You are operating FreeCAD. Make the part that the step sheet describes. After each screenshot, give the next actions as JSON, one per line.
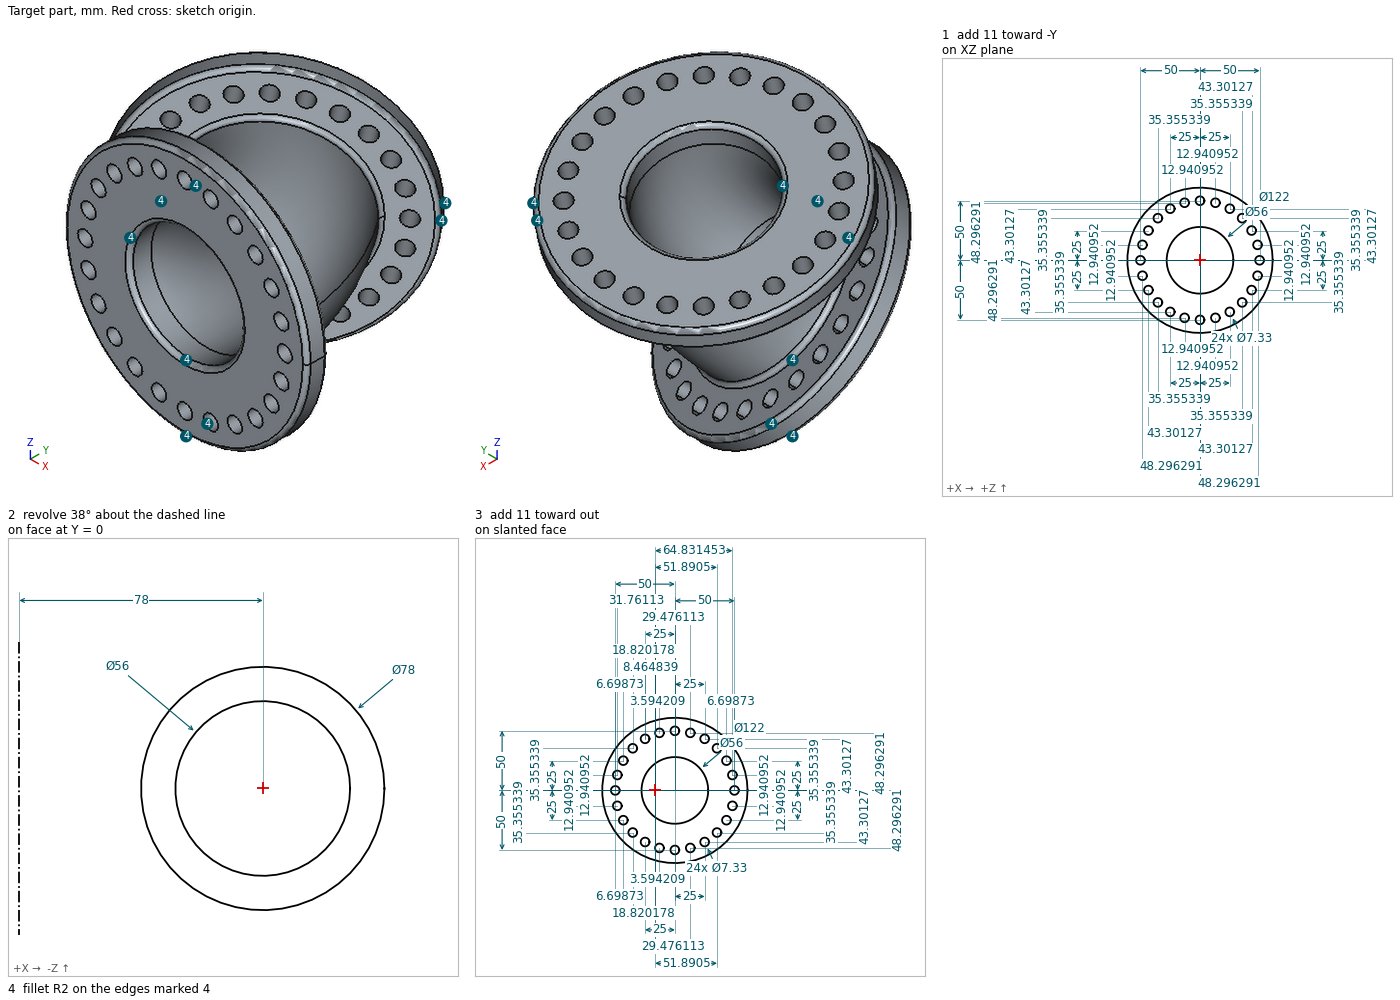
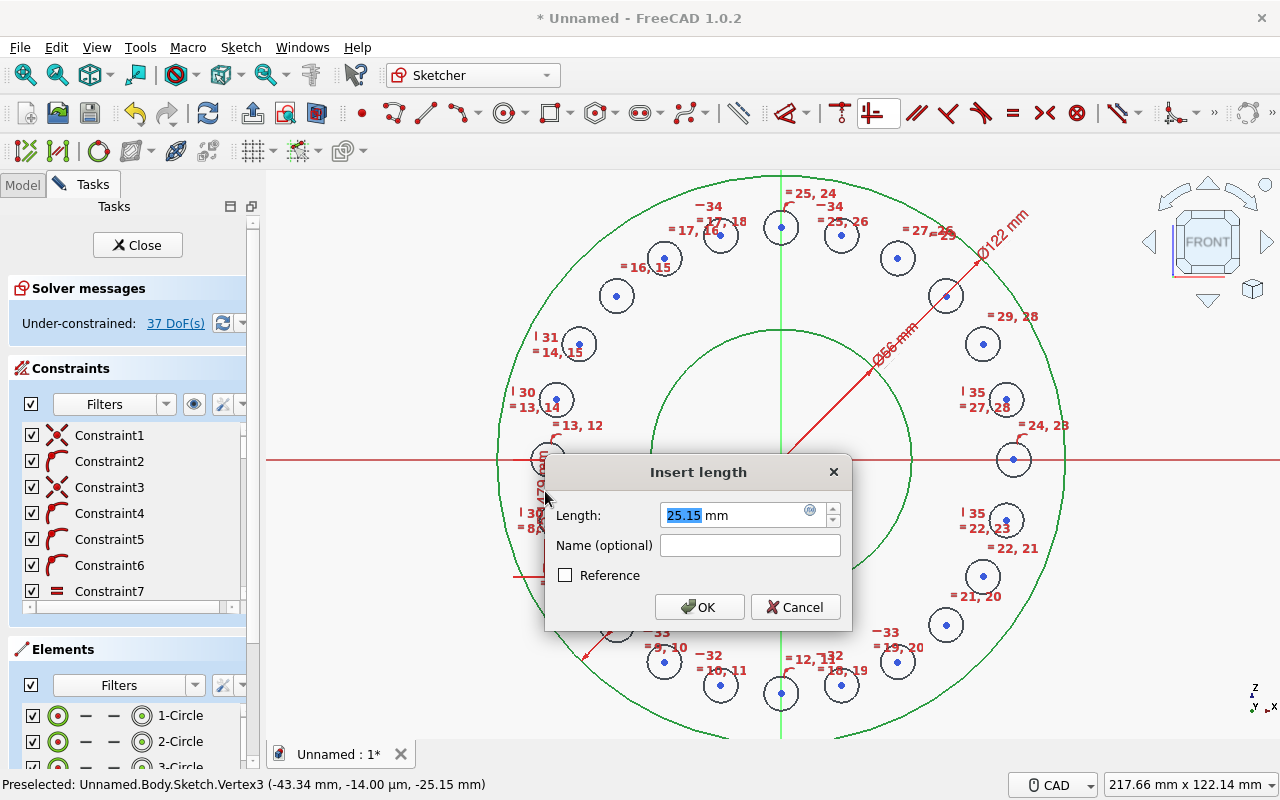
{"action": "type", "text": "25"}
{"action": "key", "text": "Return"}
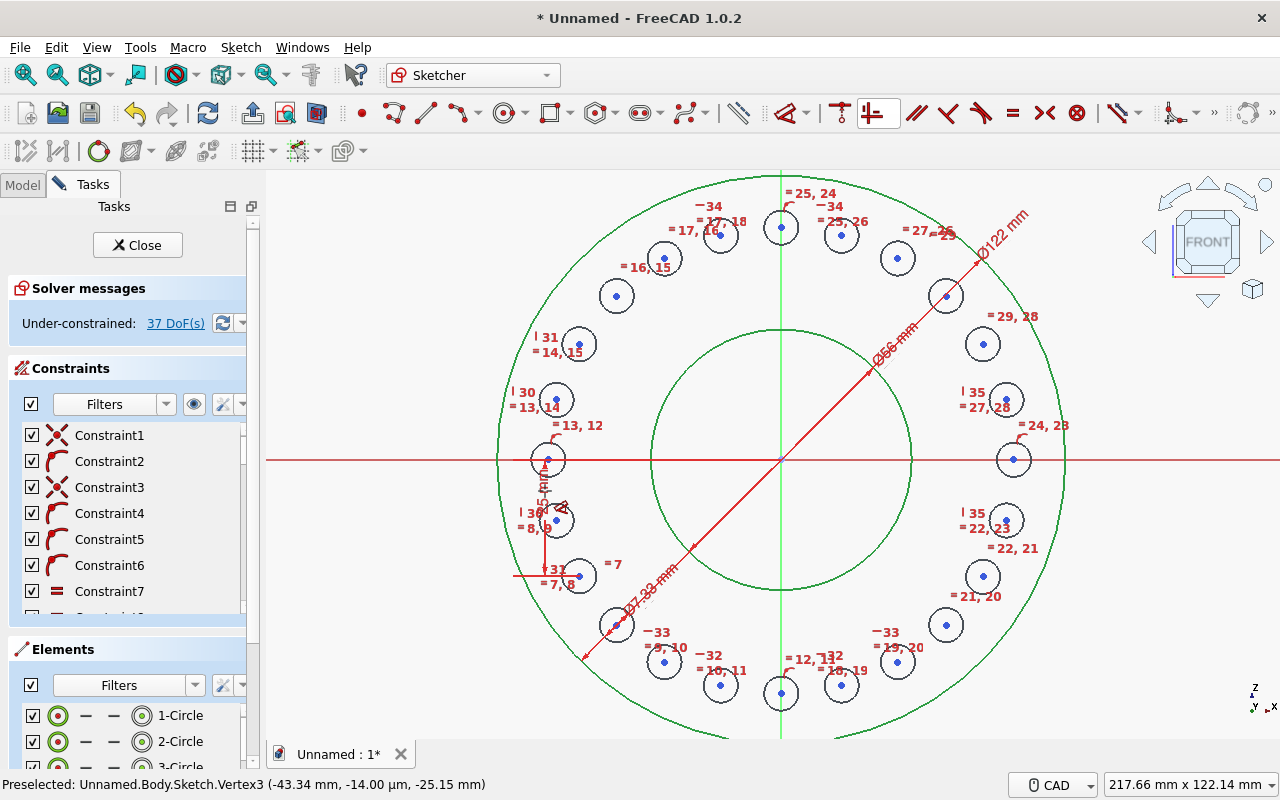
{"action": "left_click", "coordinate": [664, 662]}
{"action": "left_click", "coordinate": [750, 696]}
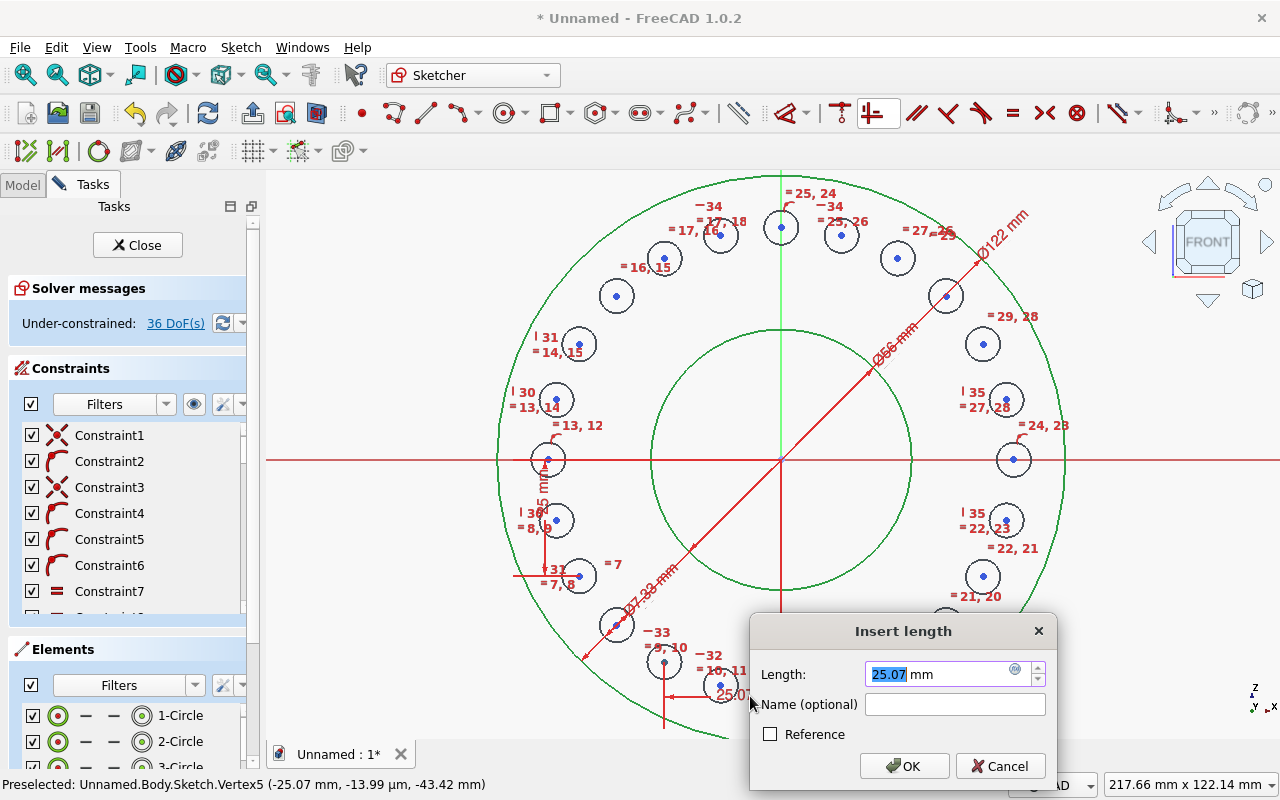
{"action": "type", "text": "25"}
{"action": "key", "text": "Return"}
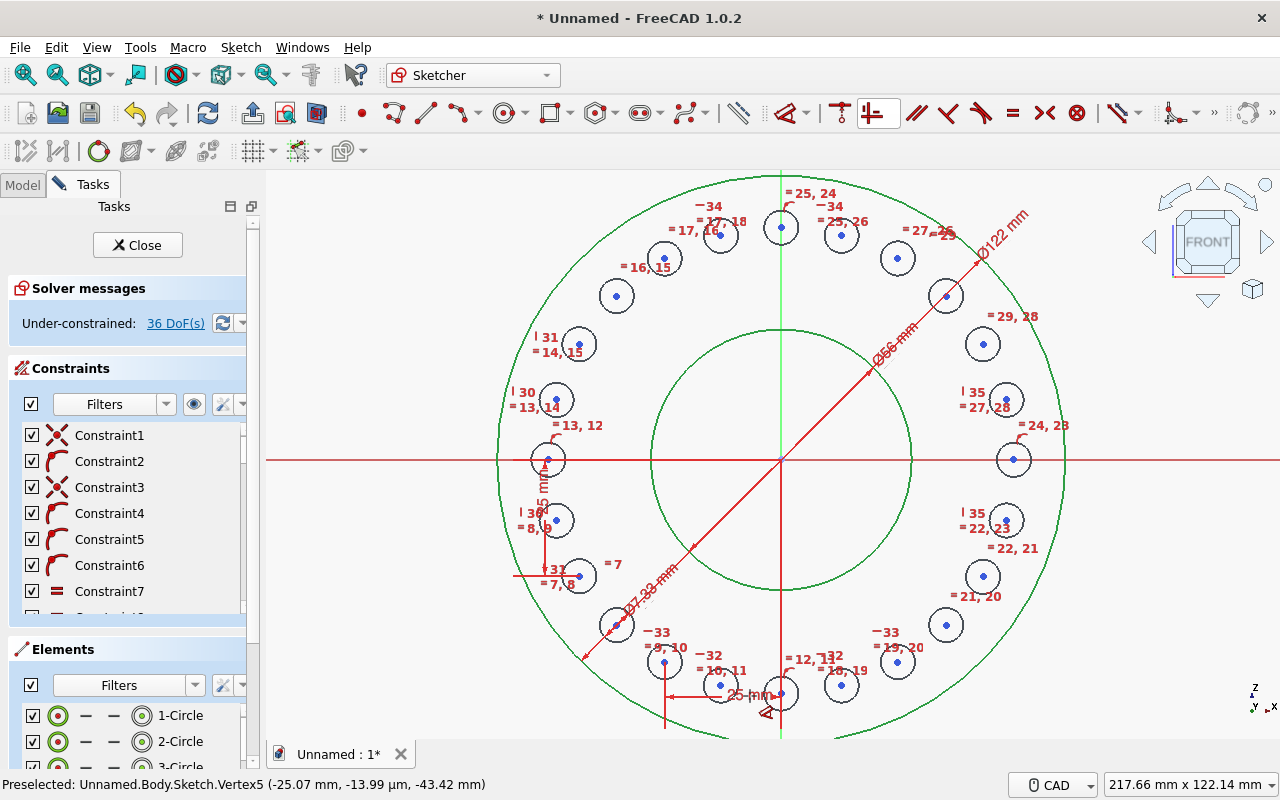
{"action": "left_click", "coordinate": [781, 694]}
{"action": "left_click", "coordinate": [815, 523]}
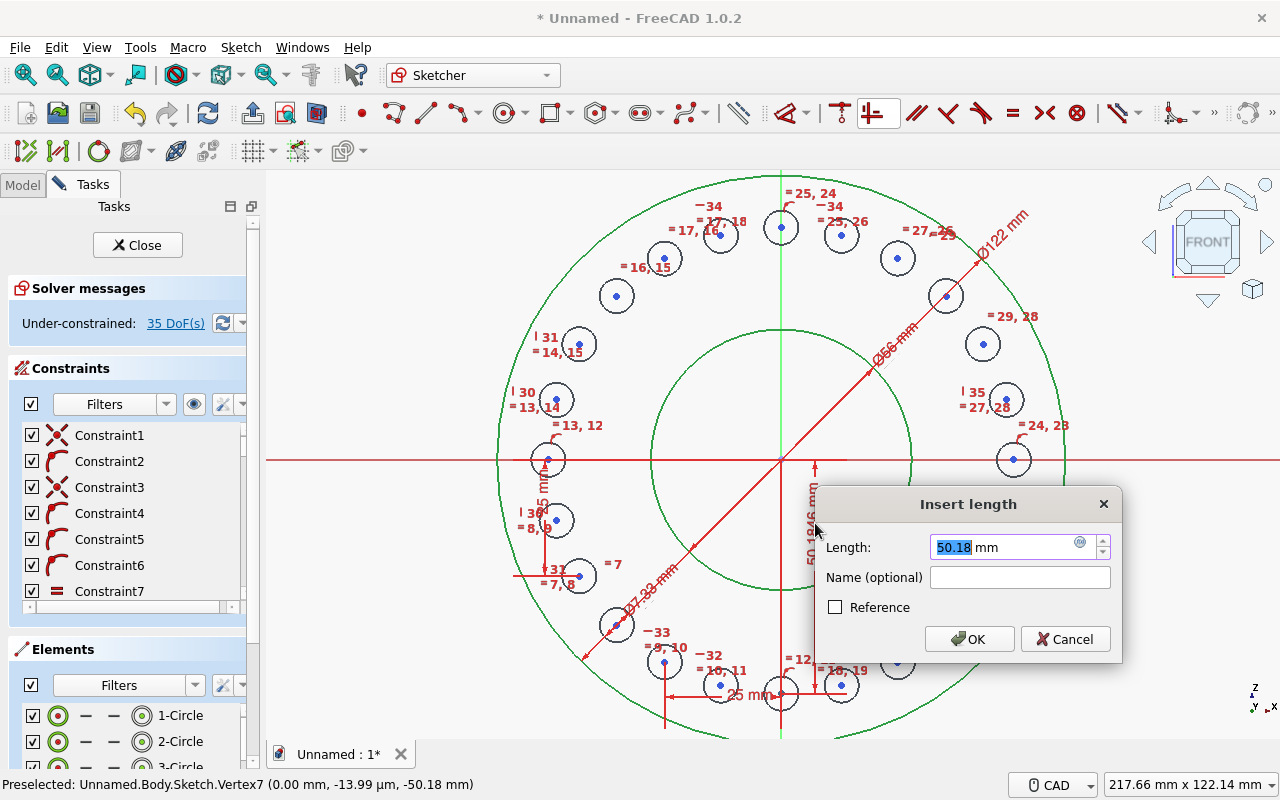
{"action": "type", "text": "50"}
{"action": "key", "text": "Return"}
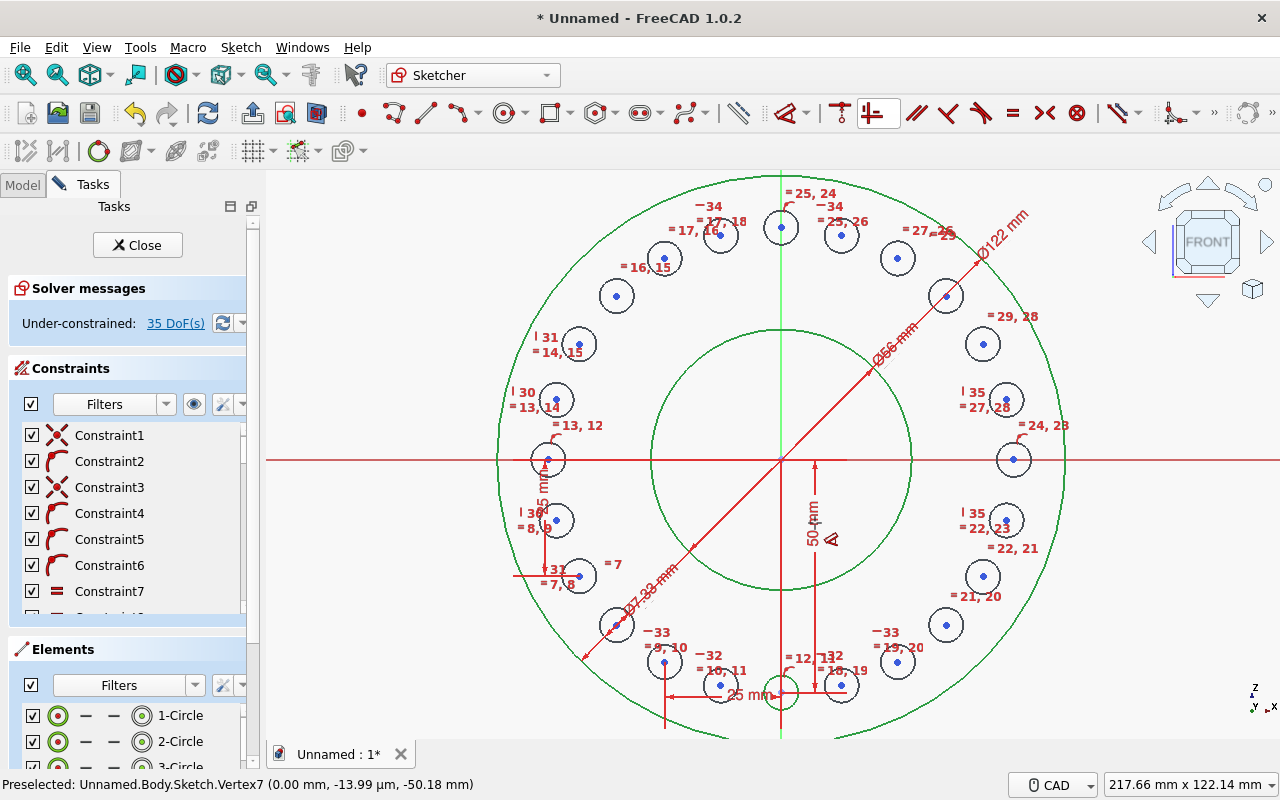
{"action": "left_click", "coordinate": [548, 460]}
{"action": "left_click", "coordinate": [718, 494]}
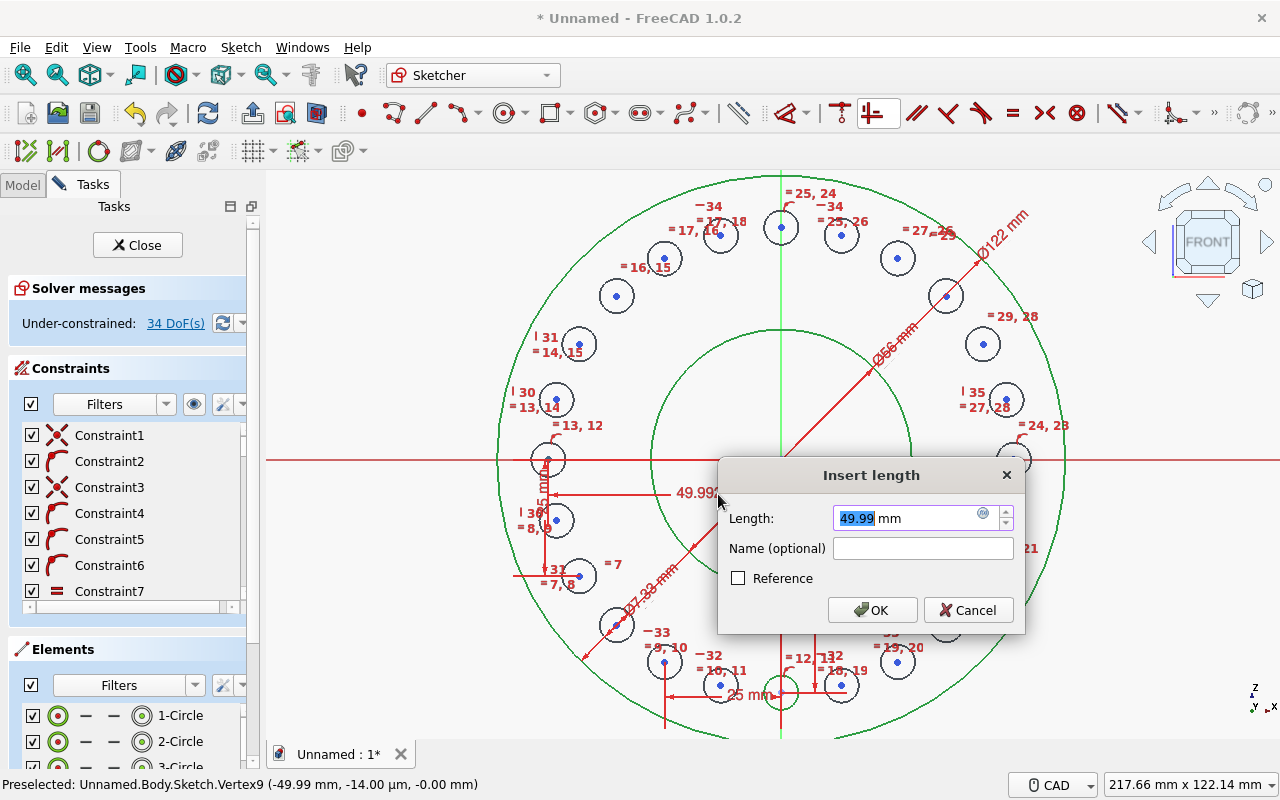
{"action": "type", "text": "50"}
{"action": "key", "text": "Return"}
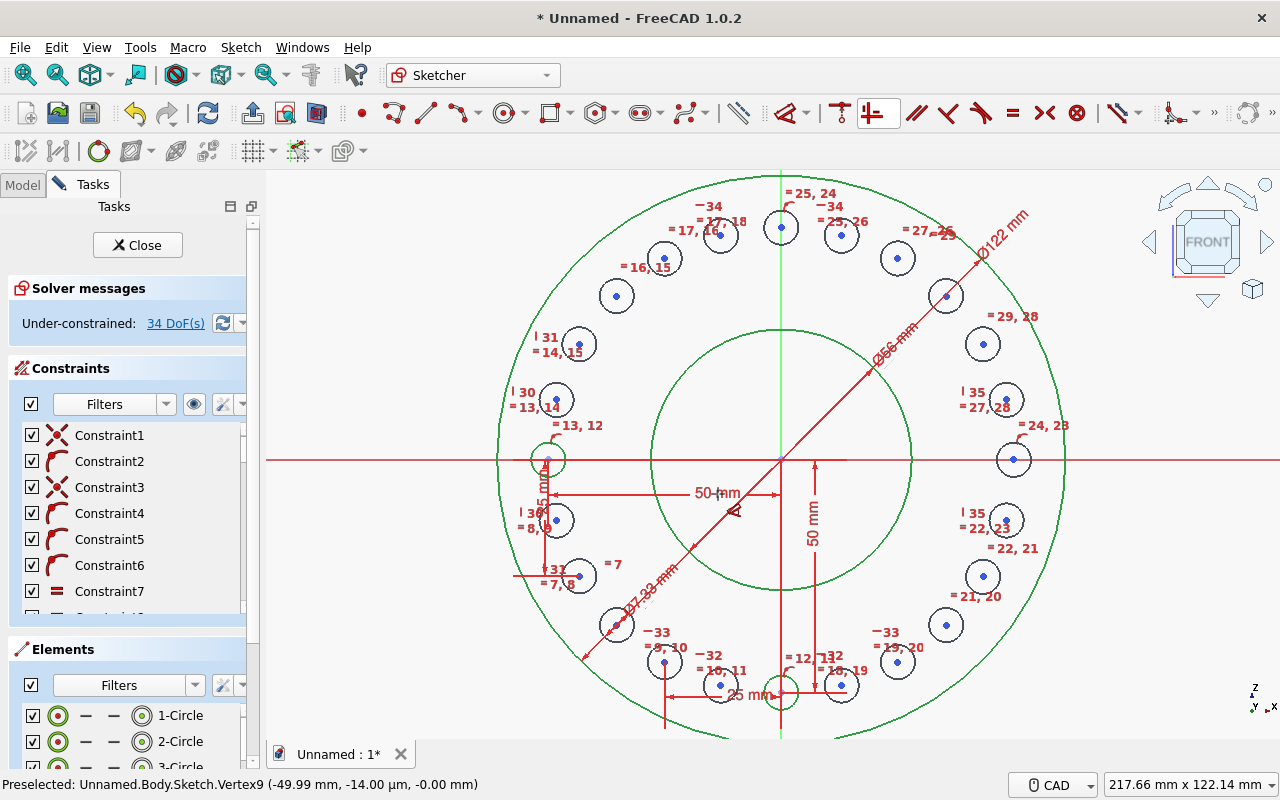
{"action": "left_click", "coordinate": [579, 344]}
{"action": "left_click", "coordinate": [545, 429]}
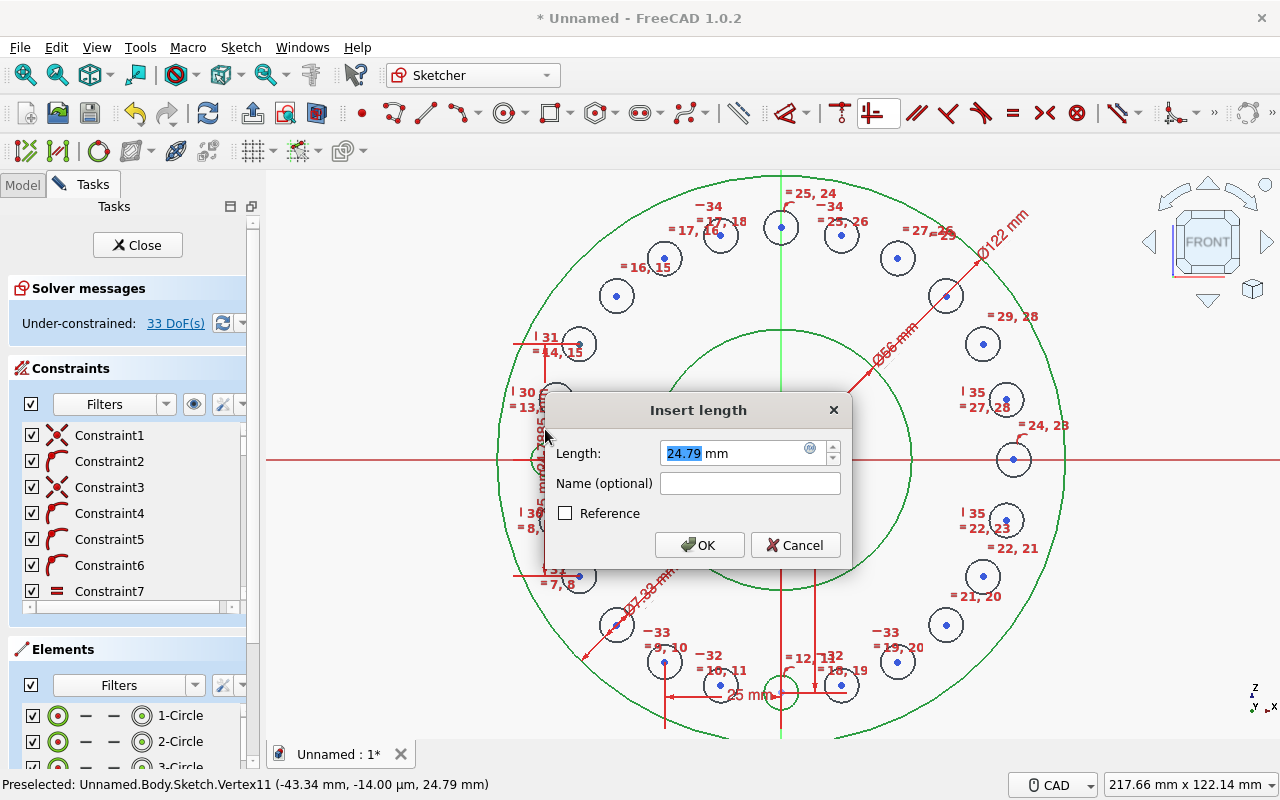
{"action": "type", "text": "25"}
{"action": "key", "text": "Return"}